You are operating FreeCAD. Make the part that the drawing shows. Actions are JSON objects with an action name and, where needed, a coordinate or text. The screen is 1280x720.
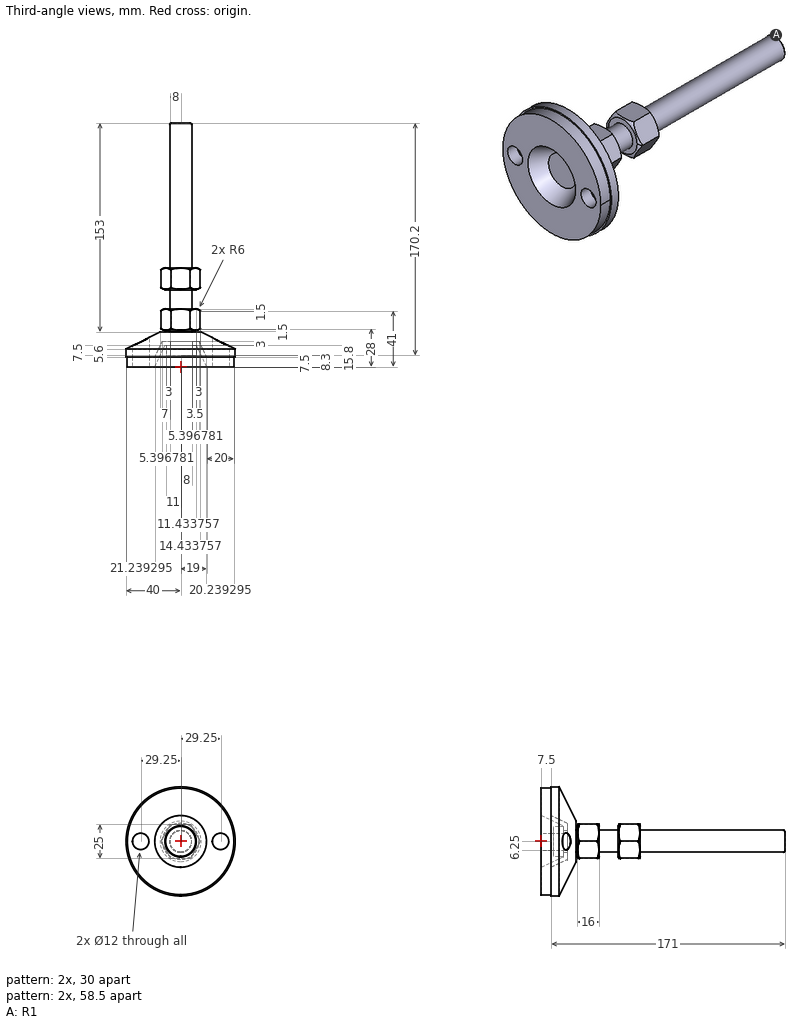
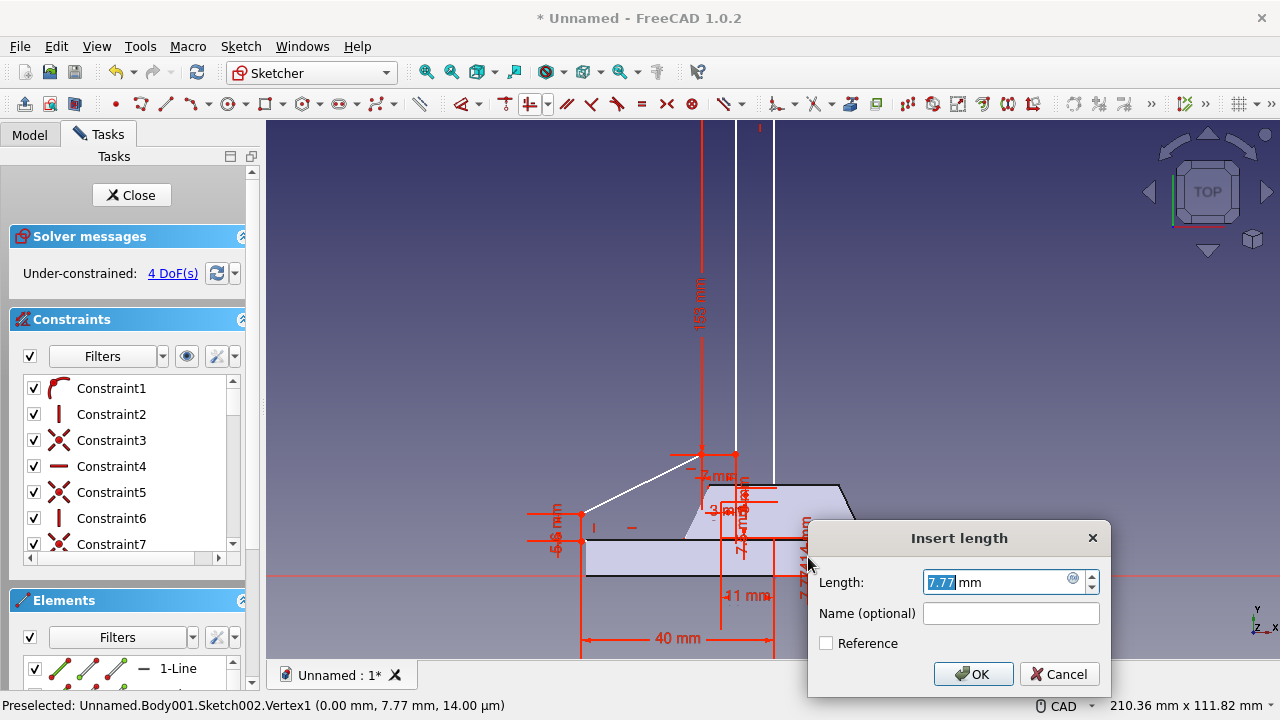
{"action": "type", "text": "8.3"}
{"action": "key", "text": "Return"}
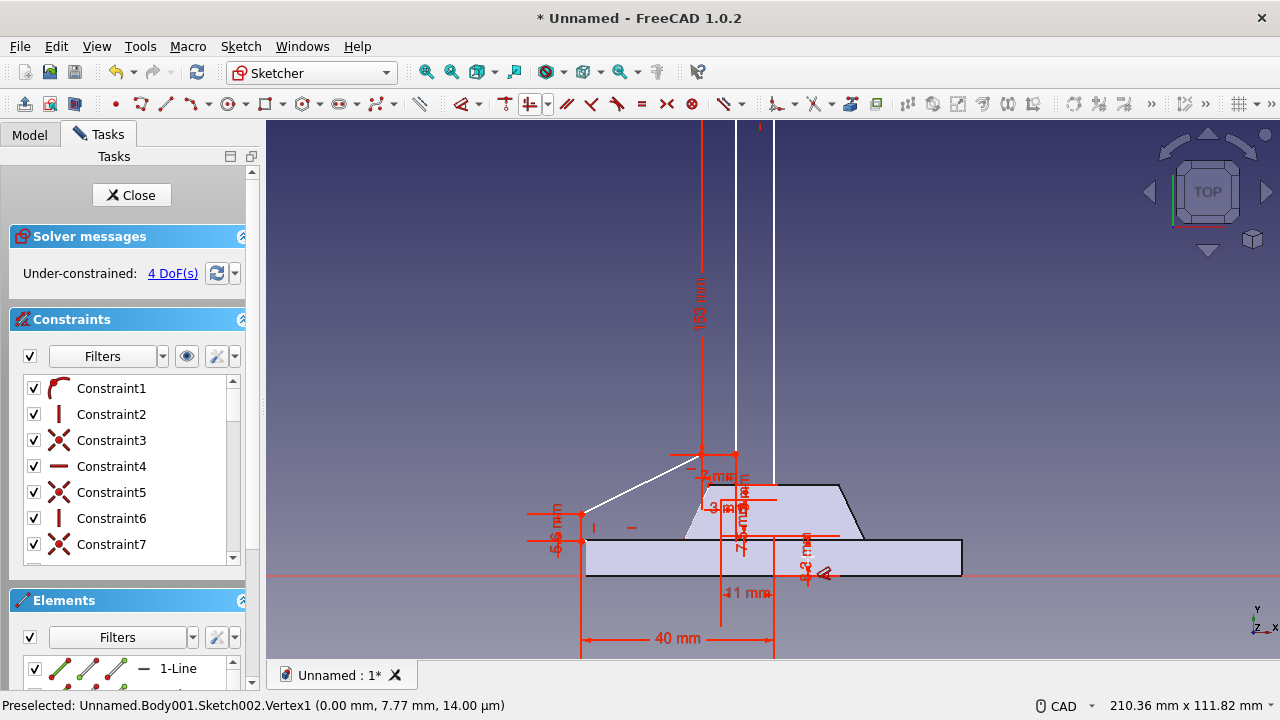
{"action": "left_click", "coordinate": [581, 541]}
{"action": "left_click", "coordinate": [547, 558]}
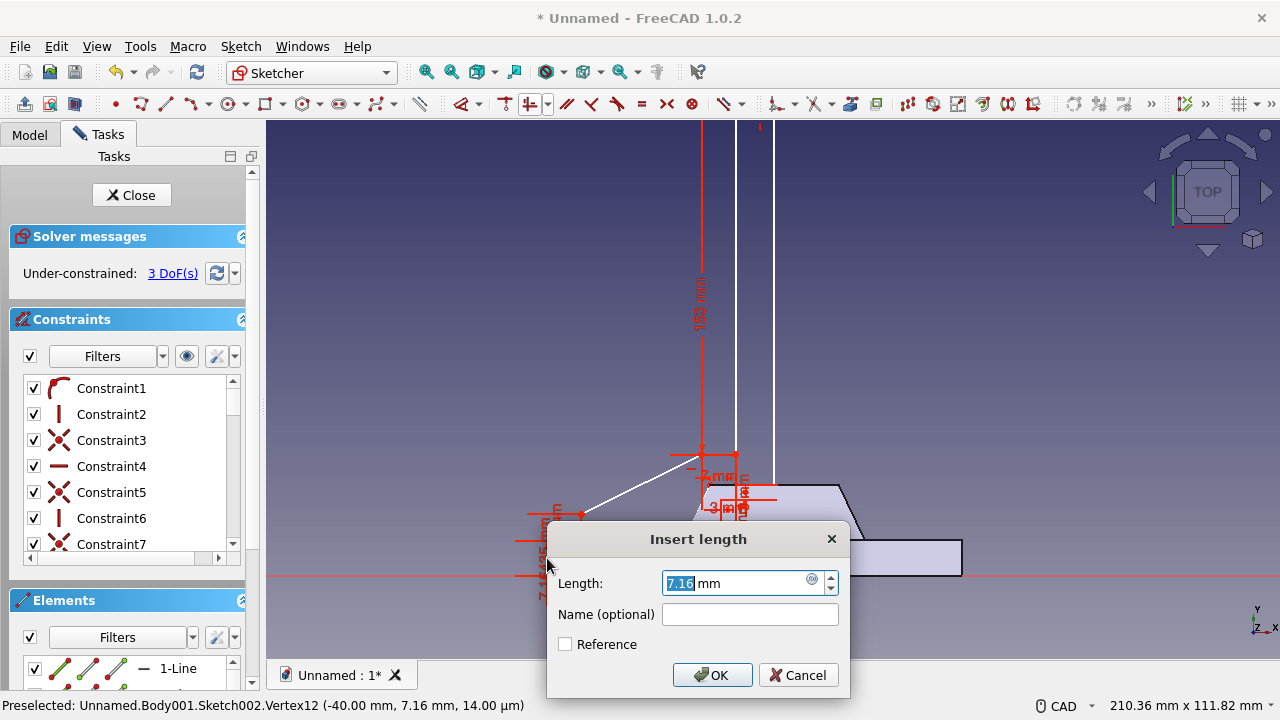
{"action": "type", "text": "7.5"}
{"action": "key", "text": "Return"}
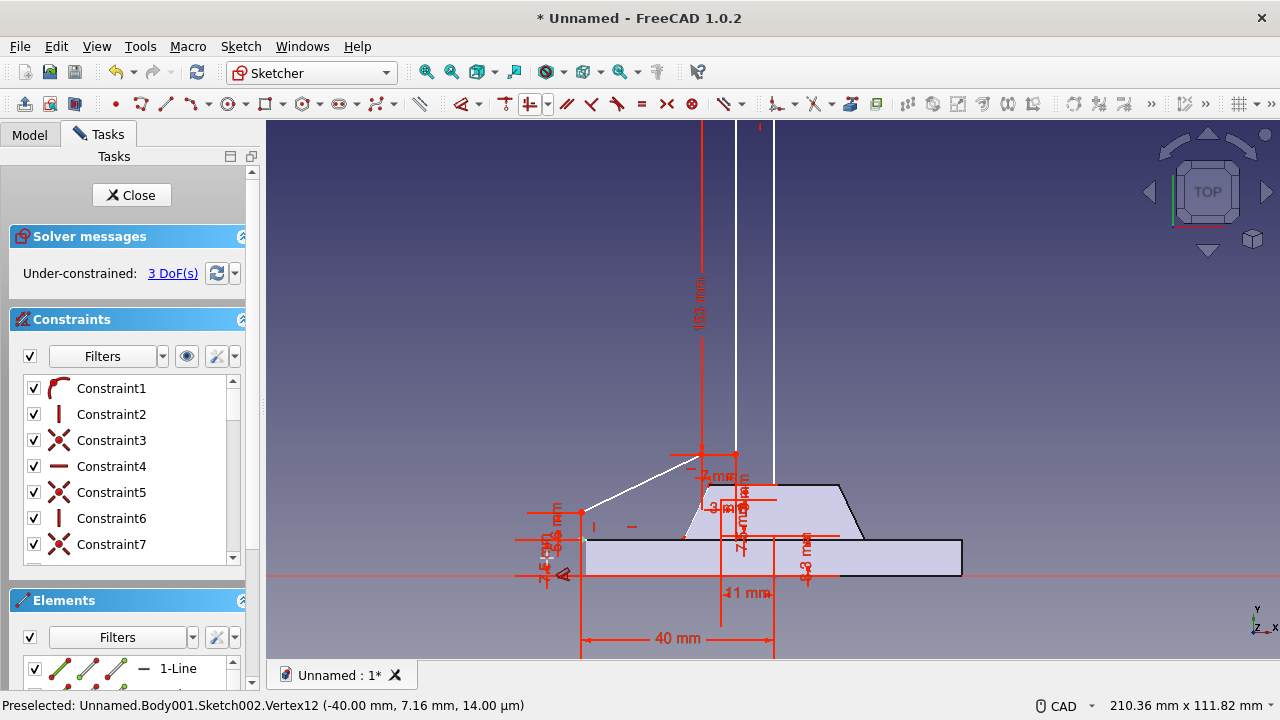
{"action": "left_click", "coordinate": [774, 290]}
{"action": "left_click", "coordinate": [808, 342]}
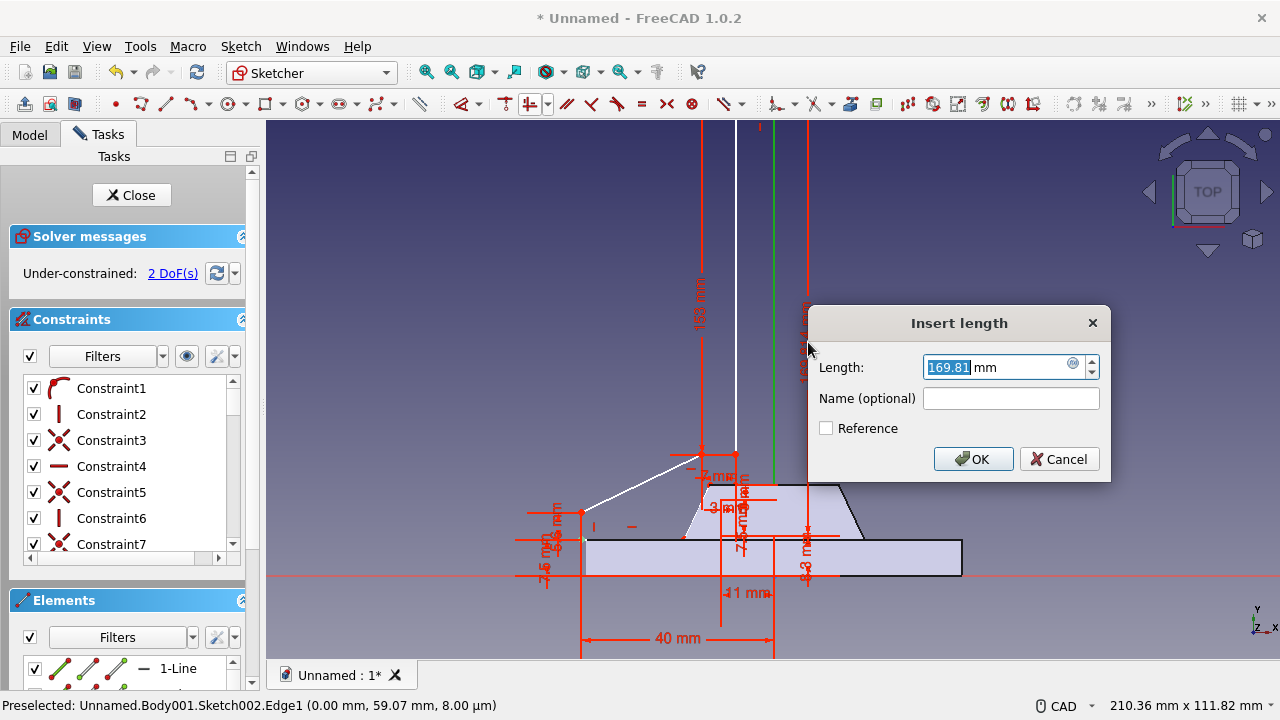
{"action": "type", "text": "170.2"}
{"action": "key", "text": "Return"}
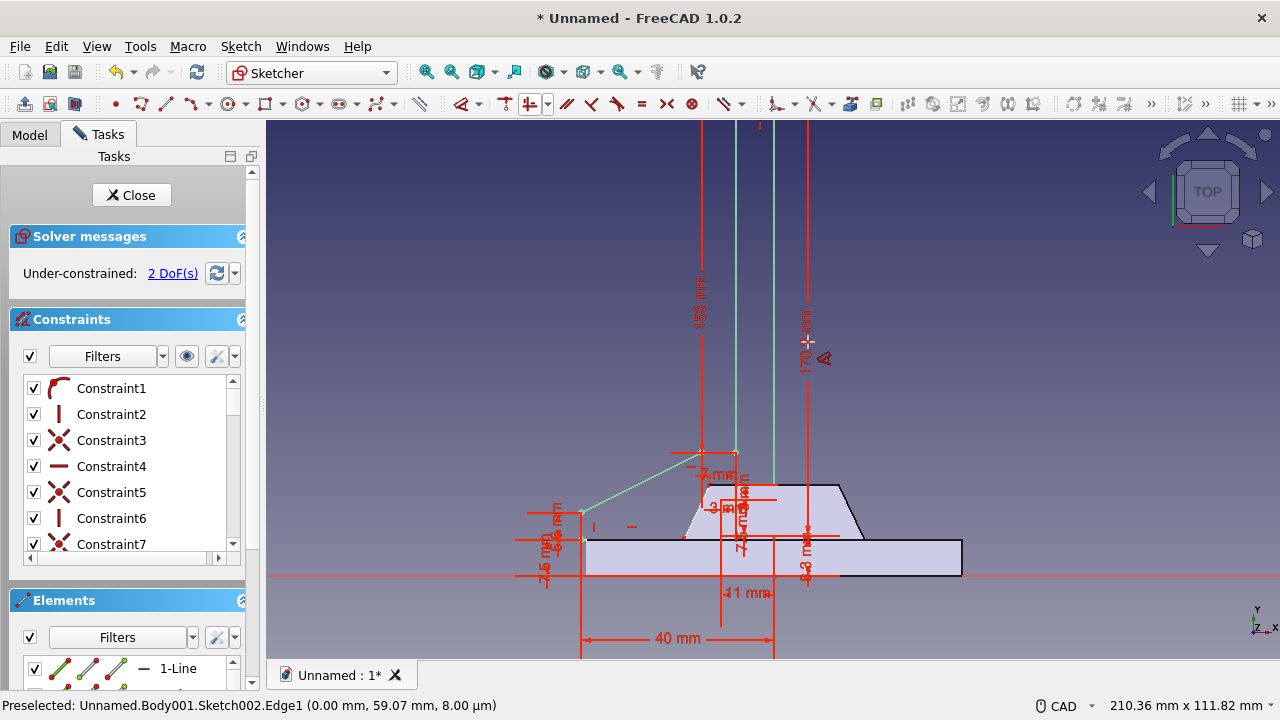
{"action": "scroll", "coordinate": [720, 485], "scroll_direction": "up", "scroll_amount": 3}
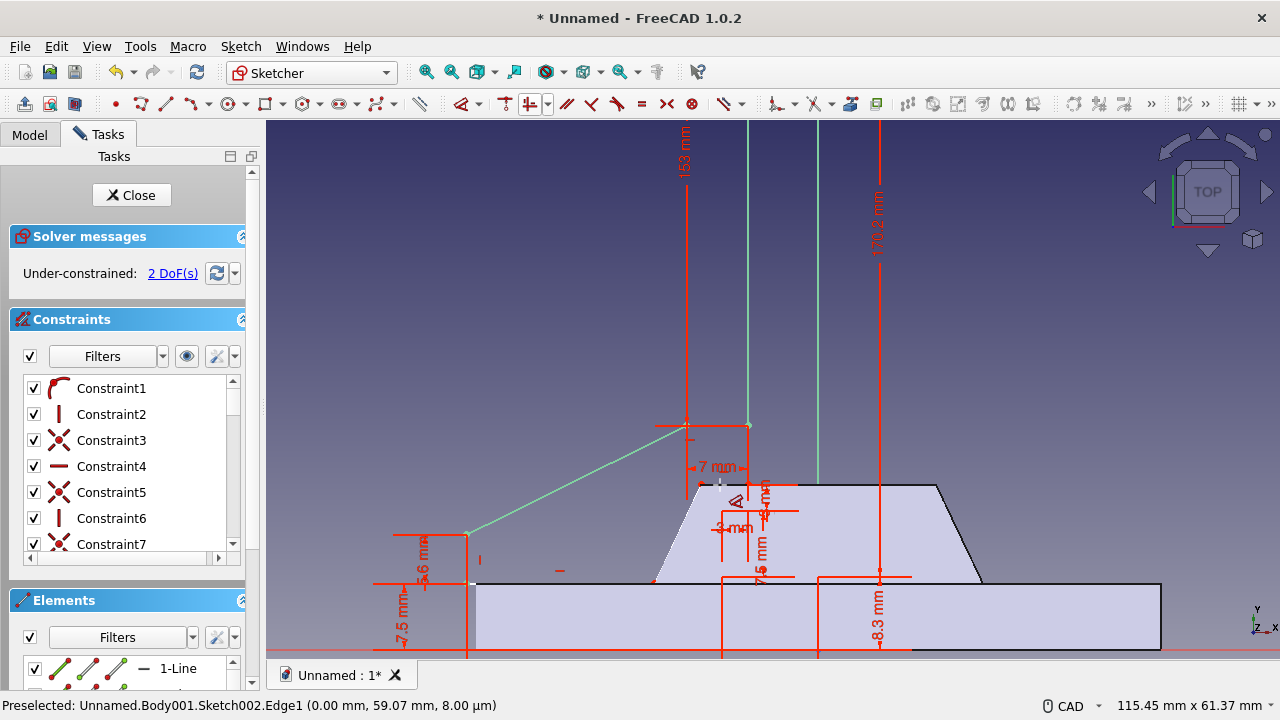
{"action": "left_click", "coordinate": [720, 485]}
{"action": "left_click", "coordinate": [725, 403]}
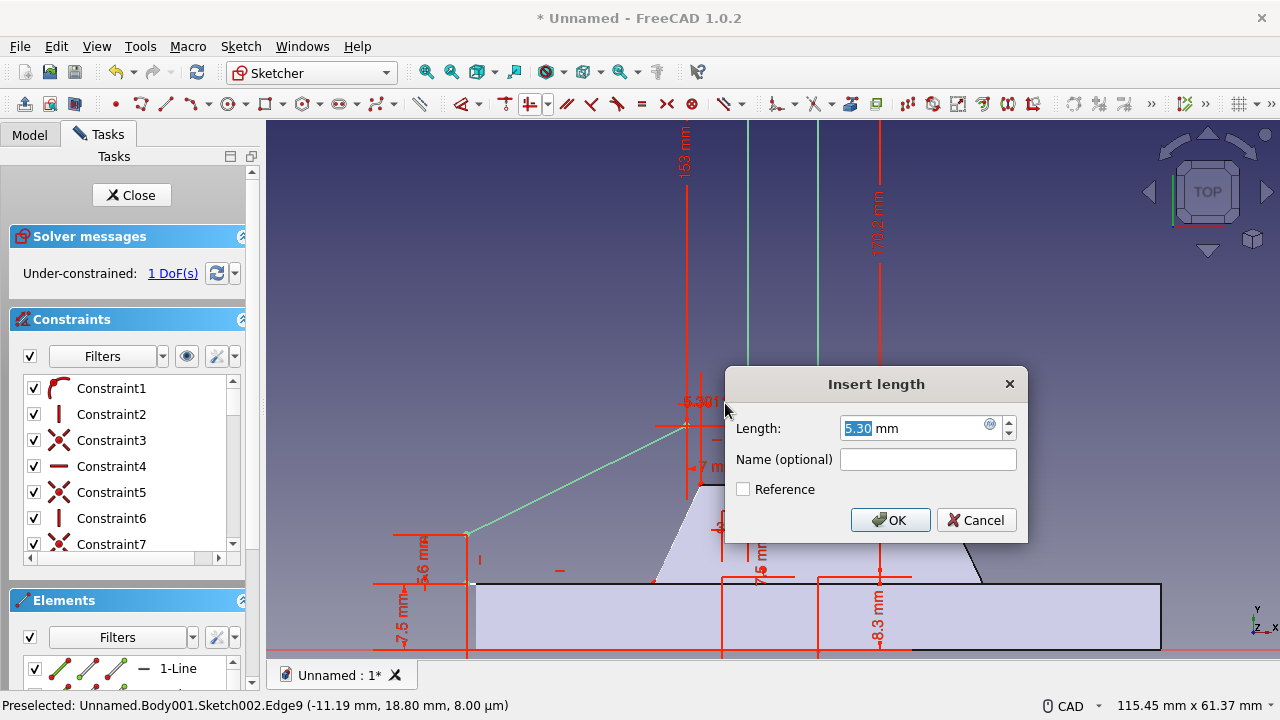
{"action": "type", "text": "5.396781"}
{"action": "key", "text": "Return"}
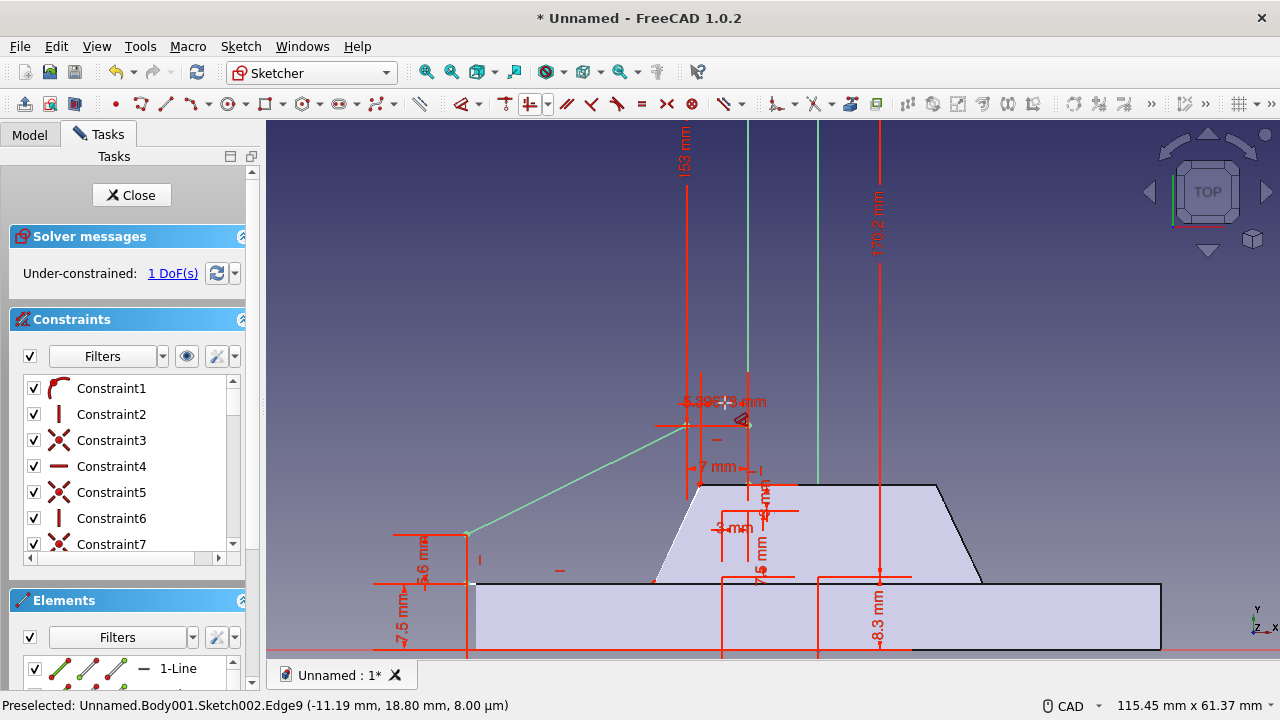
{"action": "scroll", "coordinate": [720, 522], "scroll_direction": "down", "scroll_amount": 8}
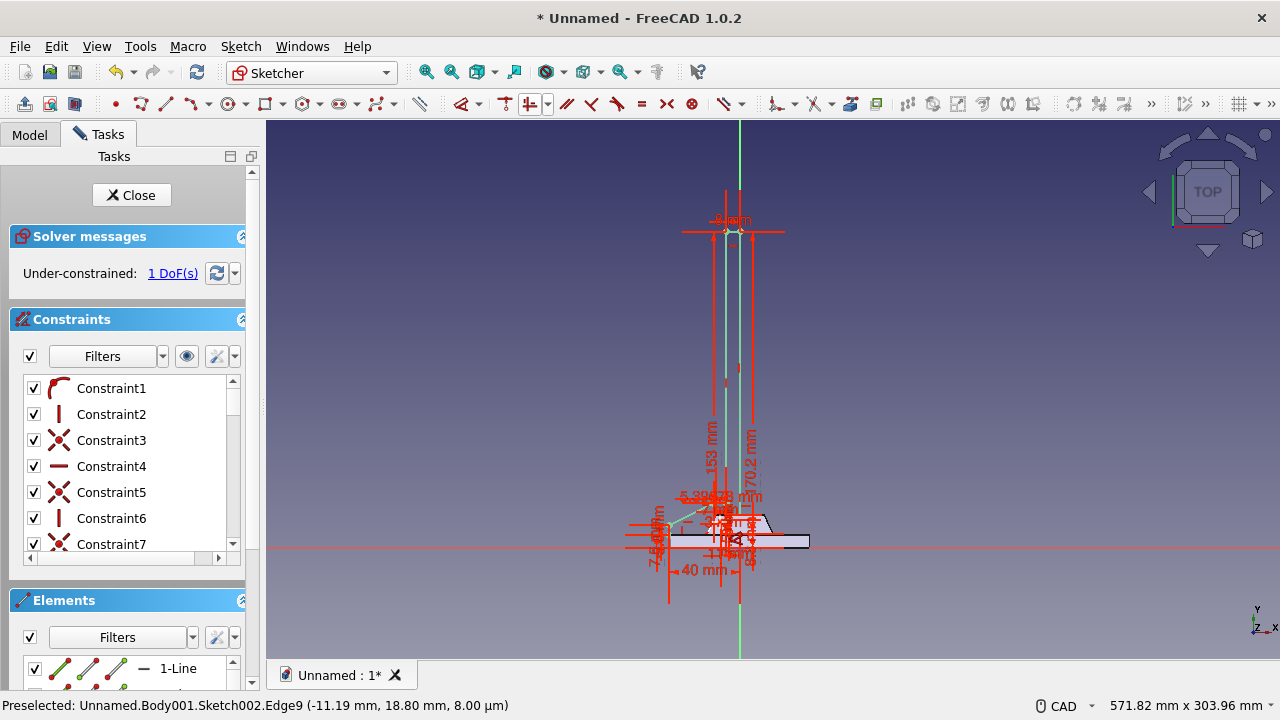
{"action": "left_click", "coordinate": [681, 535]}
{"action": "left_click", "coordinate": [688, 593]}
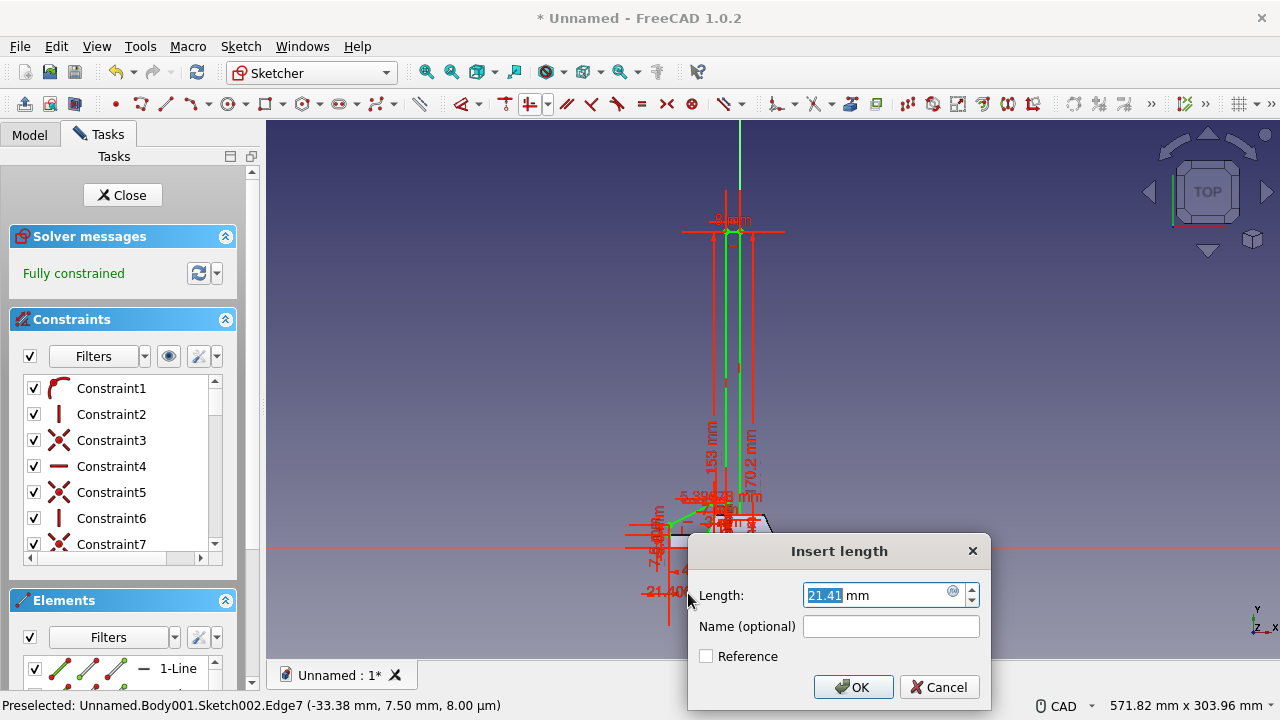
{"action": "type", "text": "21.239295"}
{"action": "key", "text": "Return"}
{"action": "key", "text": "Escape"}